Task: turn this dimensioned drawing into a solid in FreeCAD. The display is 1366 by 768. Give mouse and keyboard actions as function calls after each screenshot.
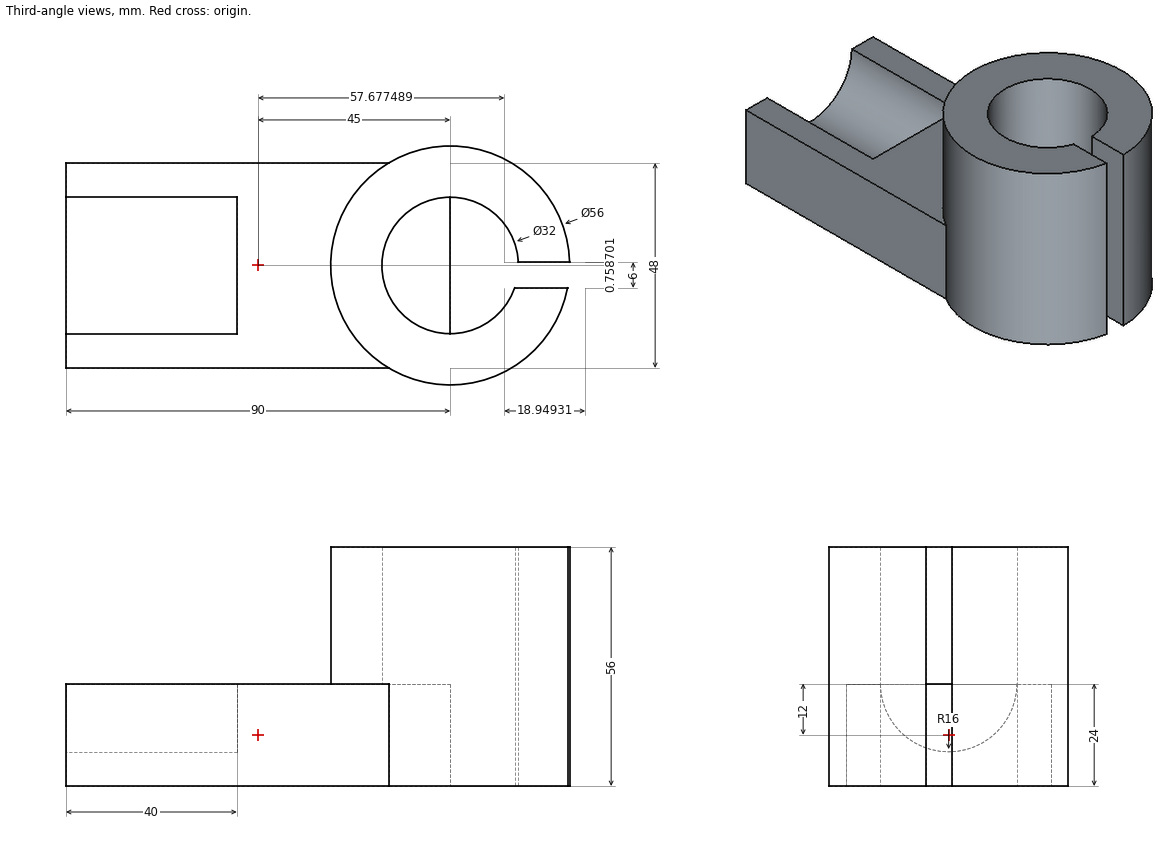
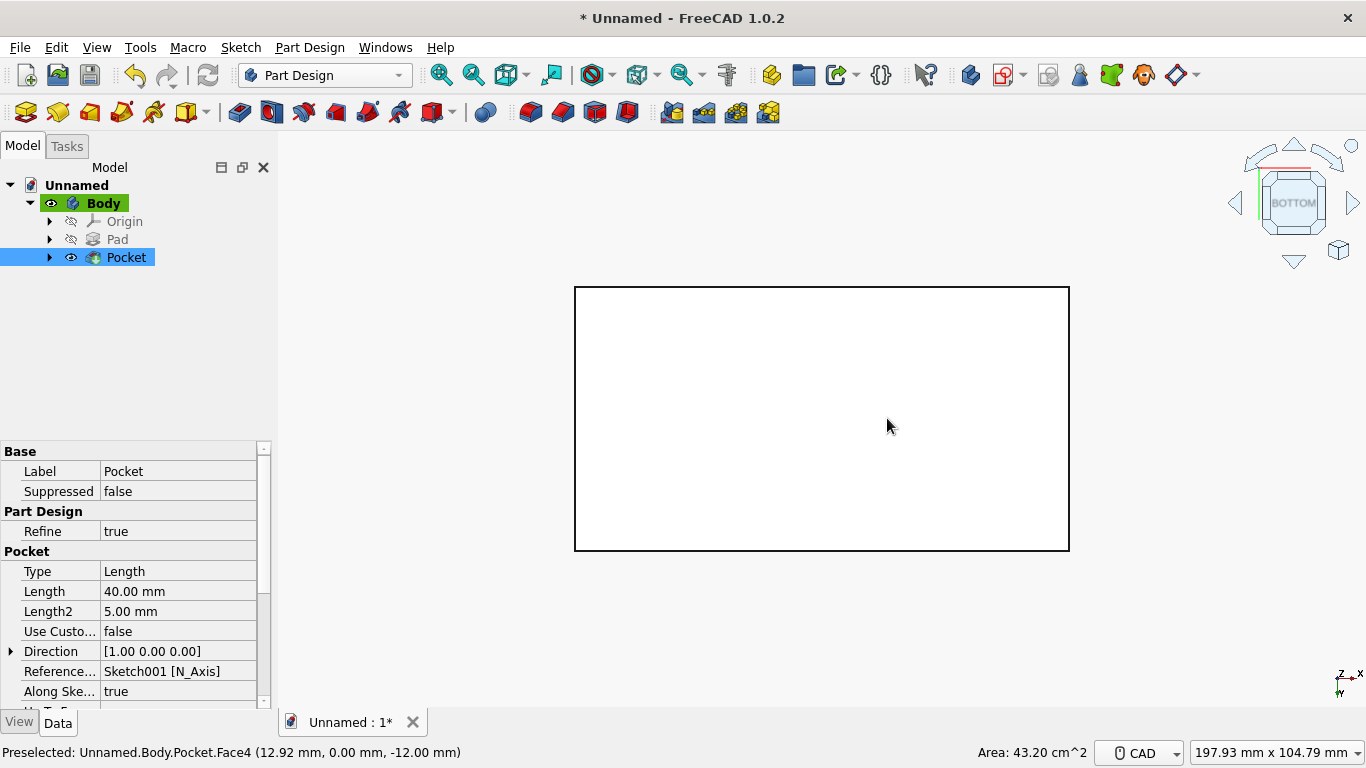
click(1004, 76)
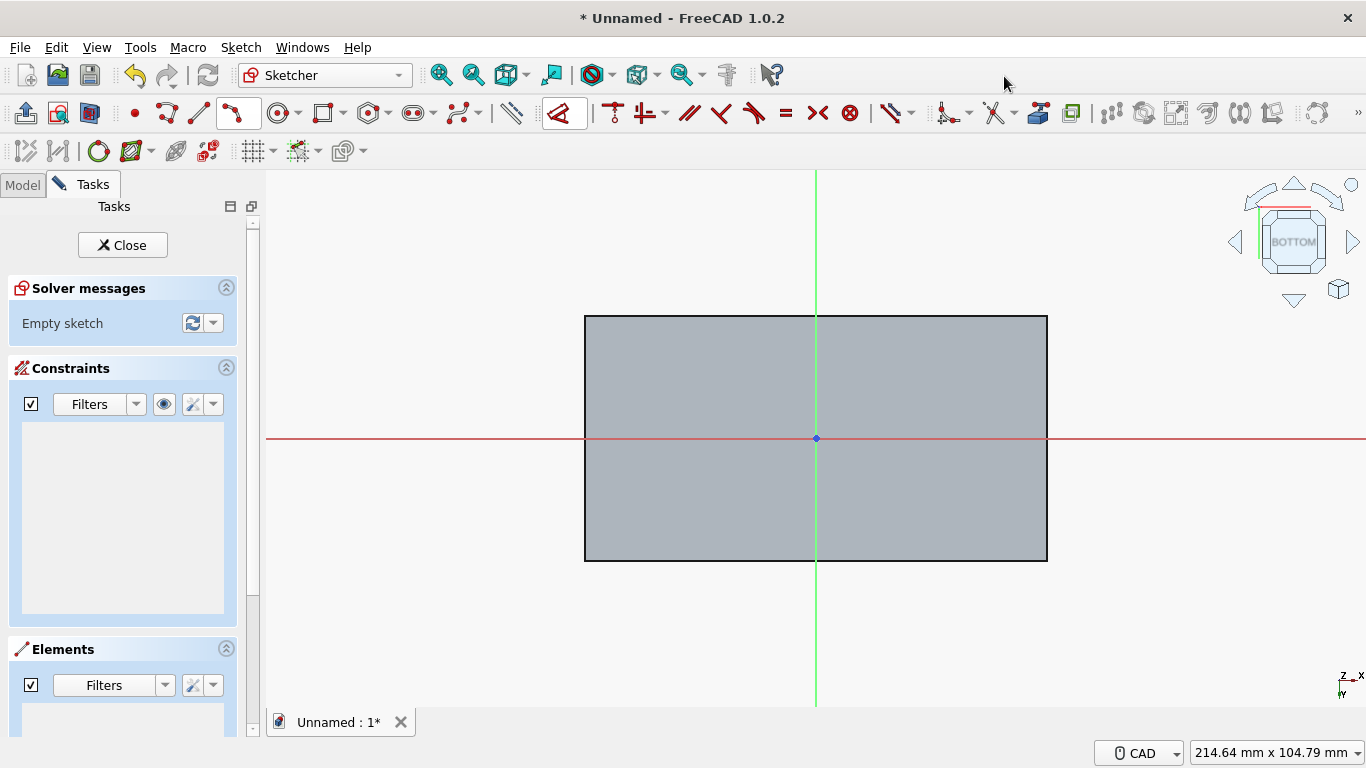
scroll(294, 439, down, 1)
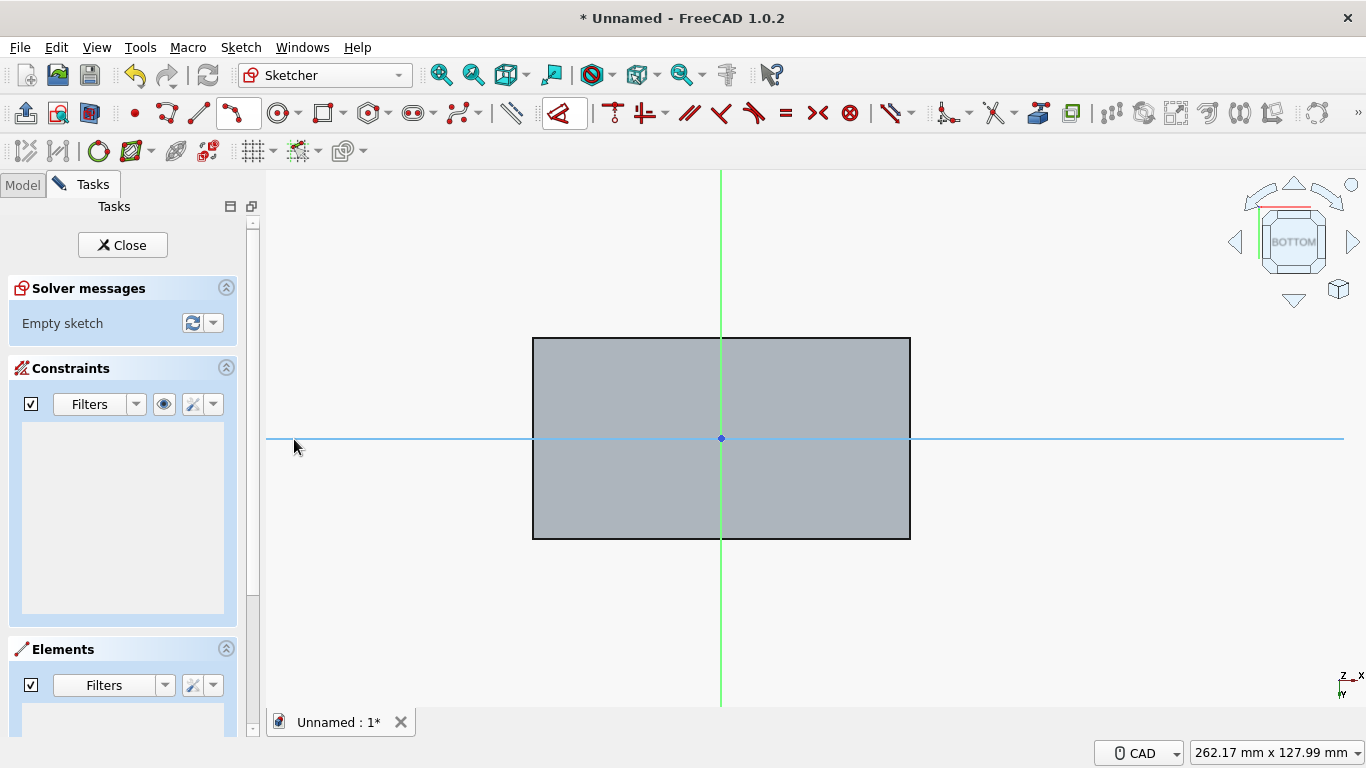
scroll(1133, 439, up, 2)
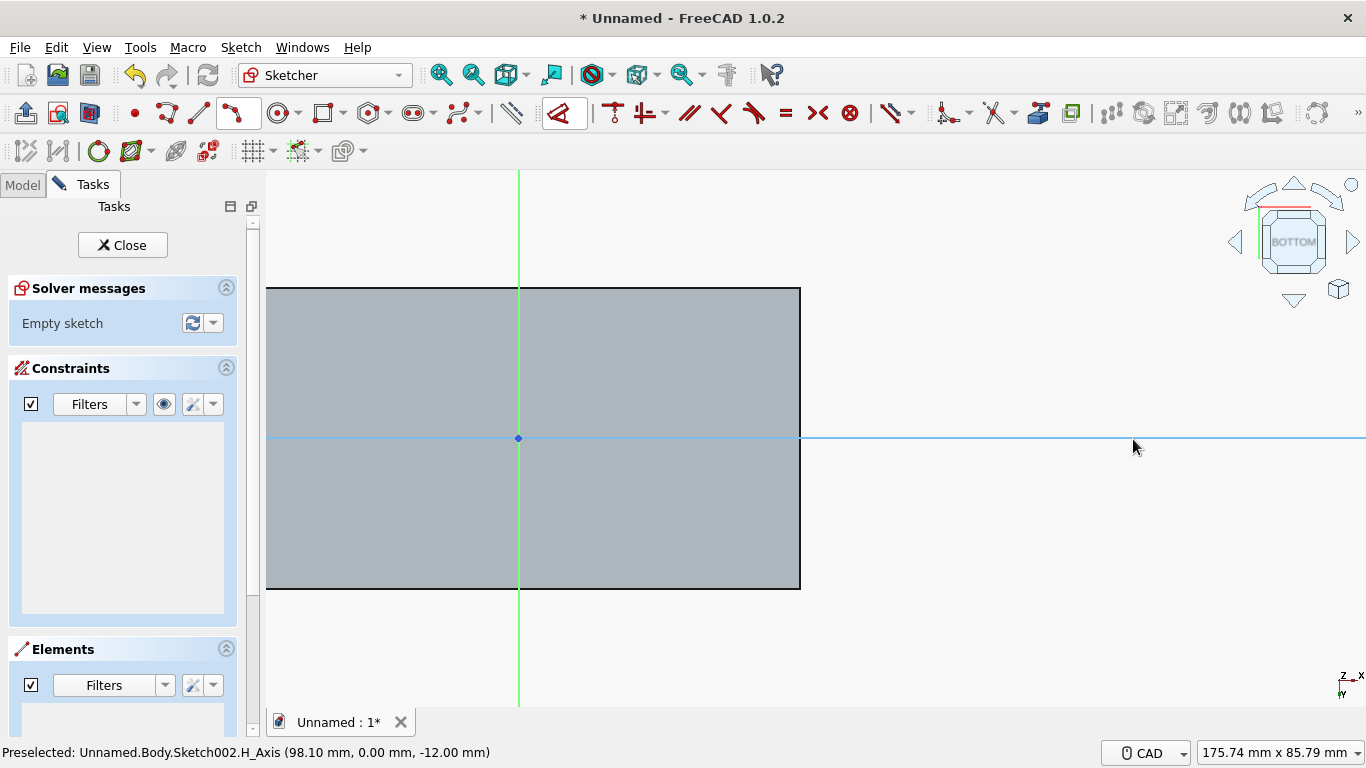
key(g)
key(c)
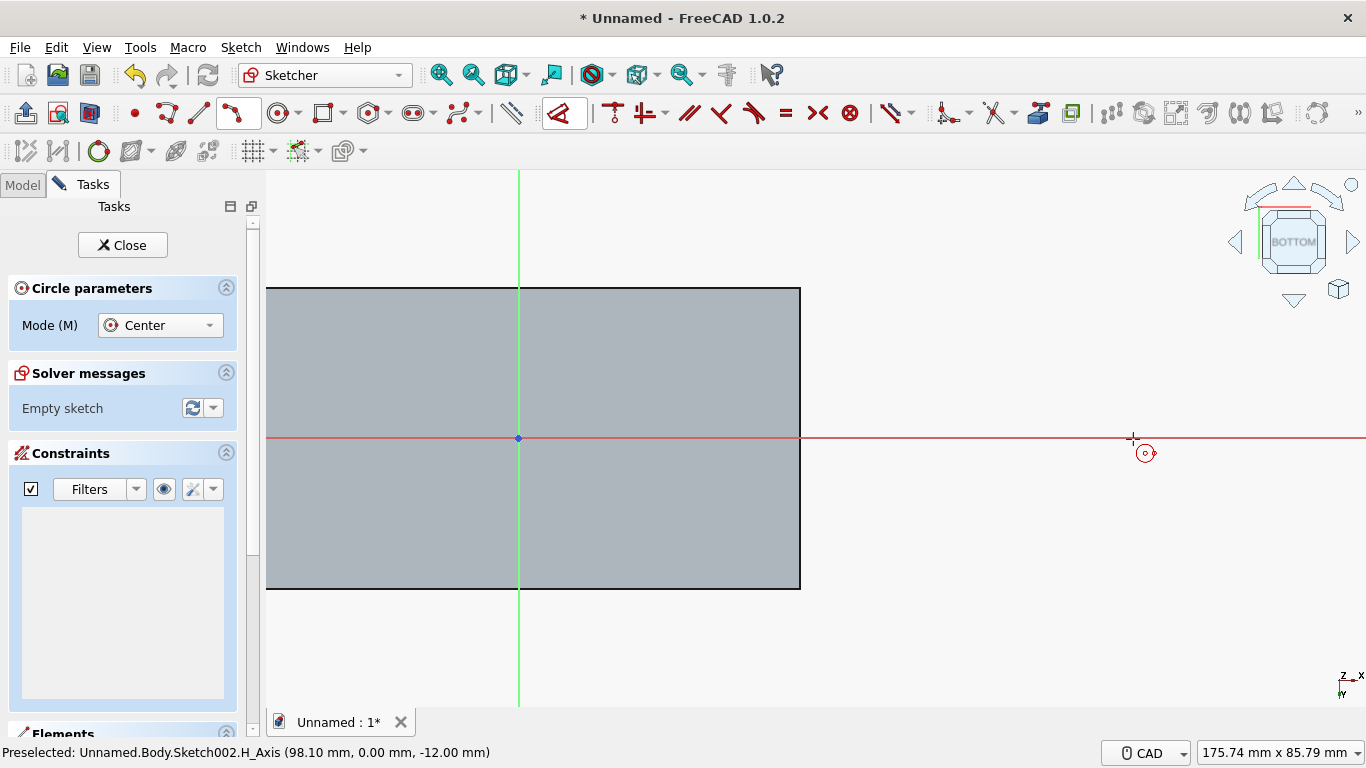
click(800, 438)
move(924, 314)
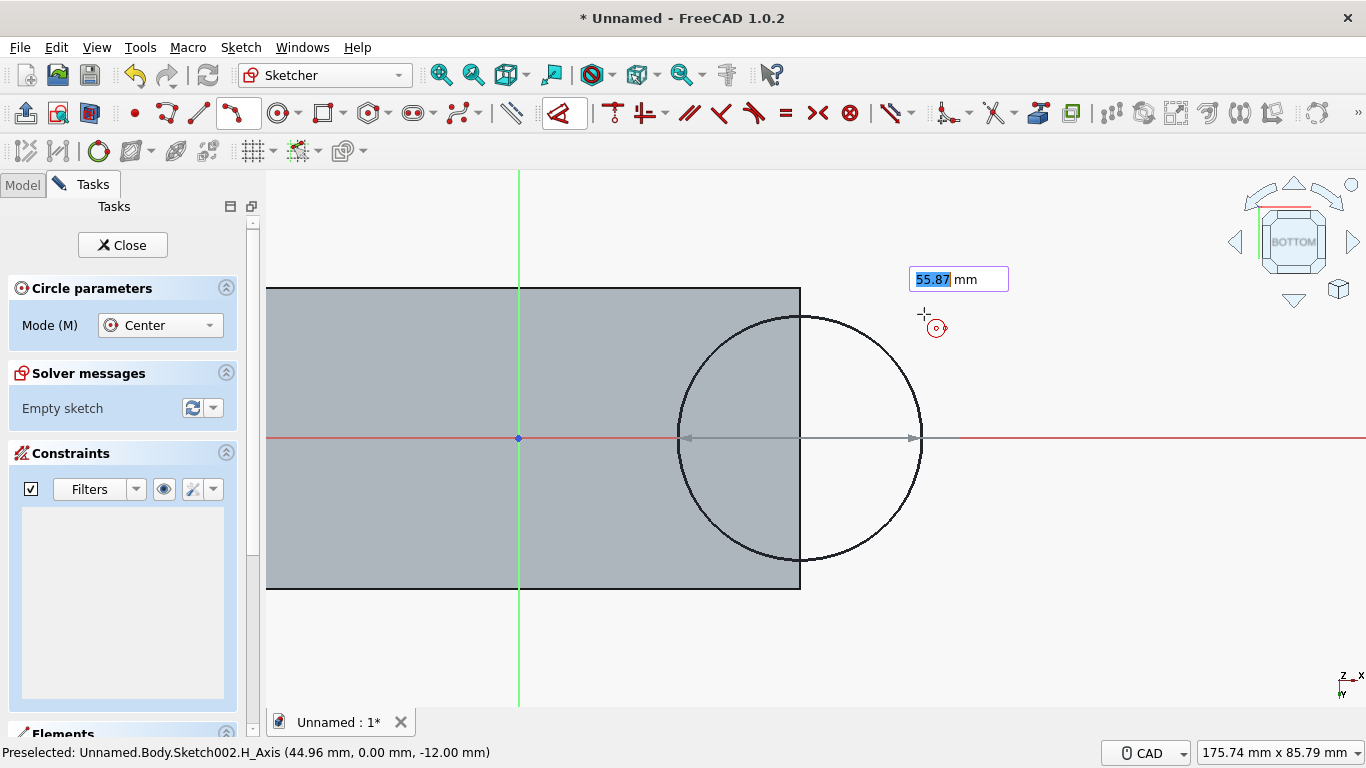
text(56)
key(Return)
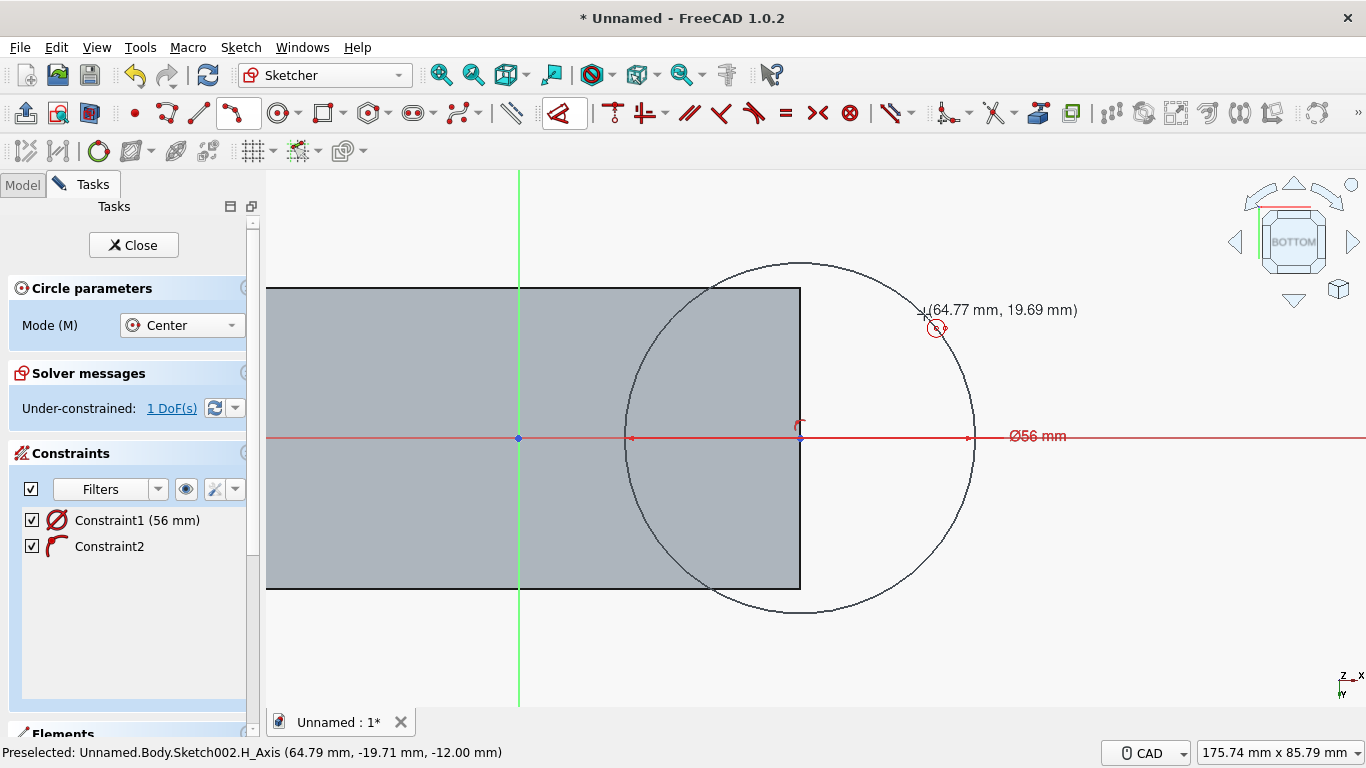
click(800, 438)
move(871, 367)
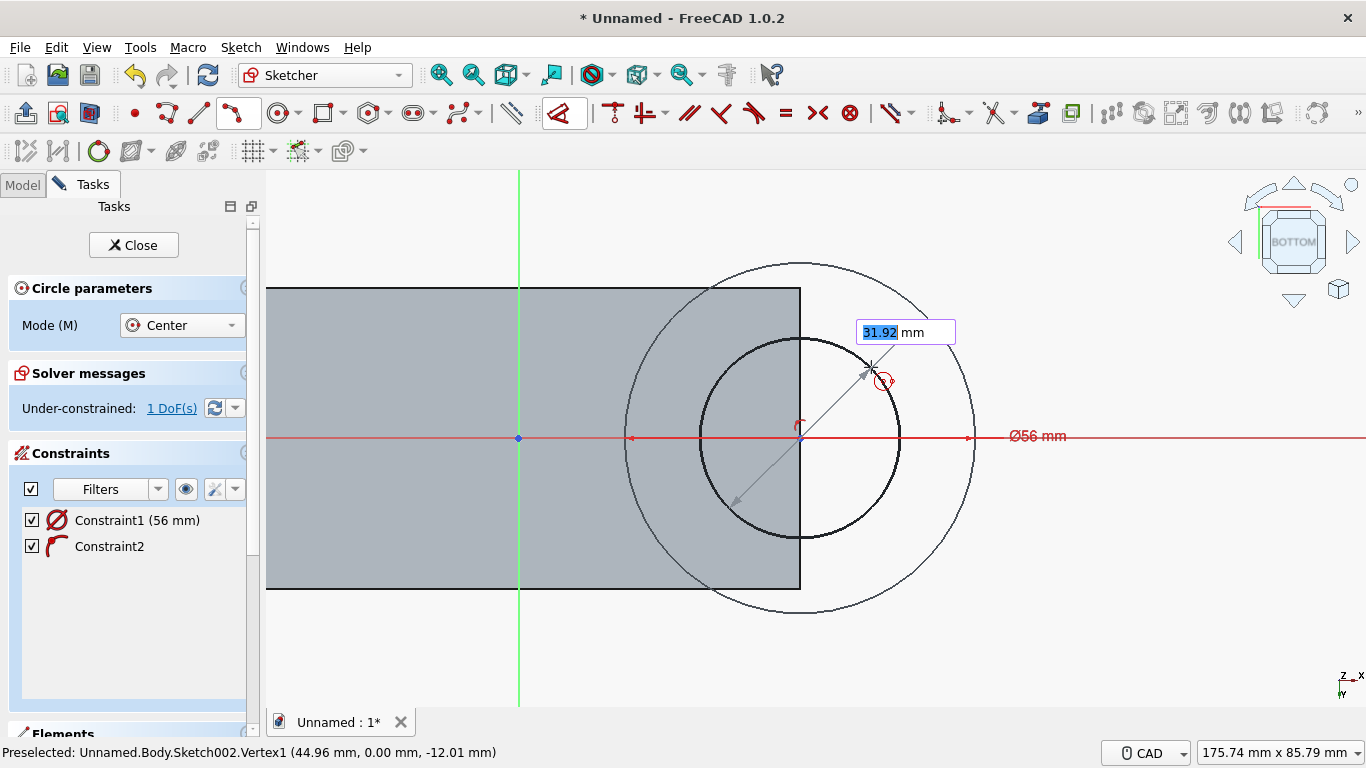
text(32)
key(Return)
key(Escape)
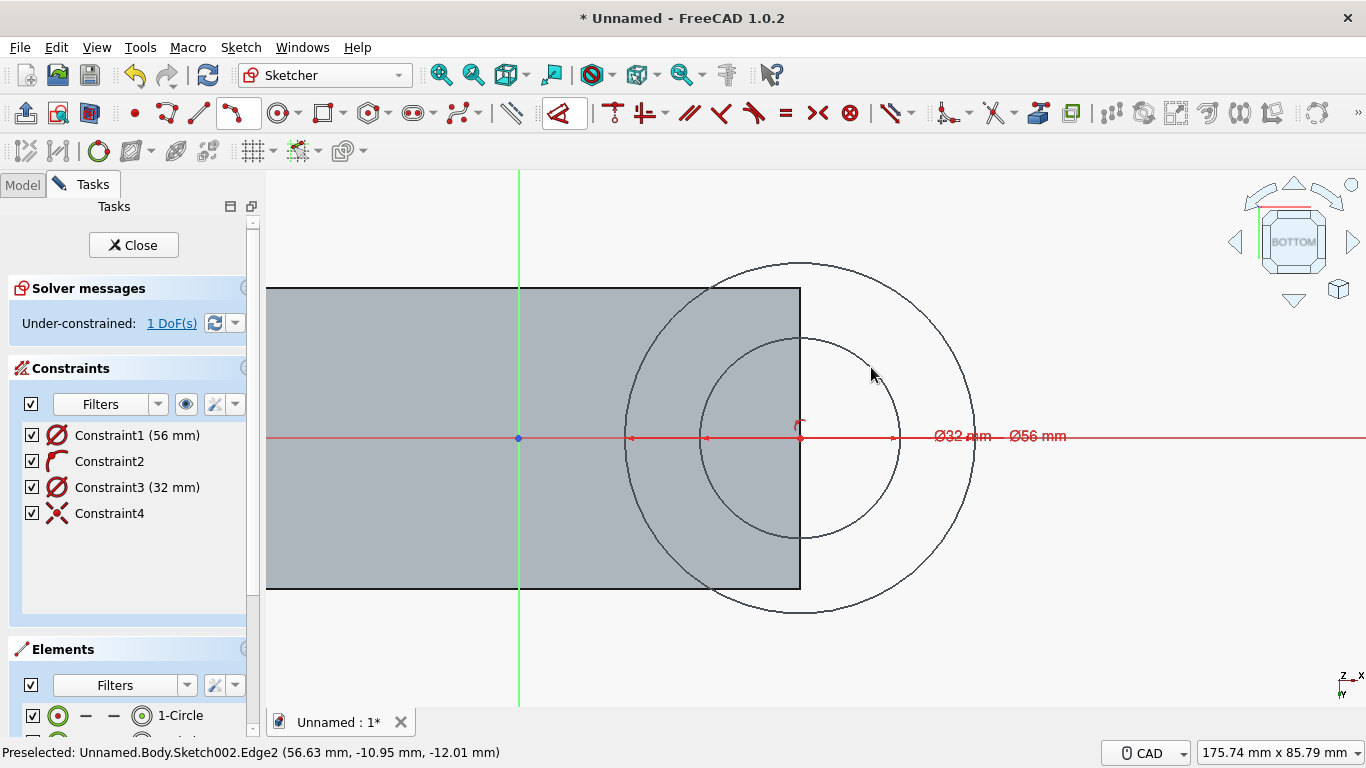
key(d)